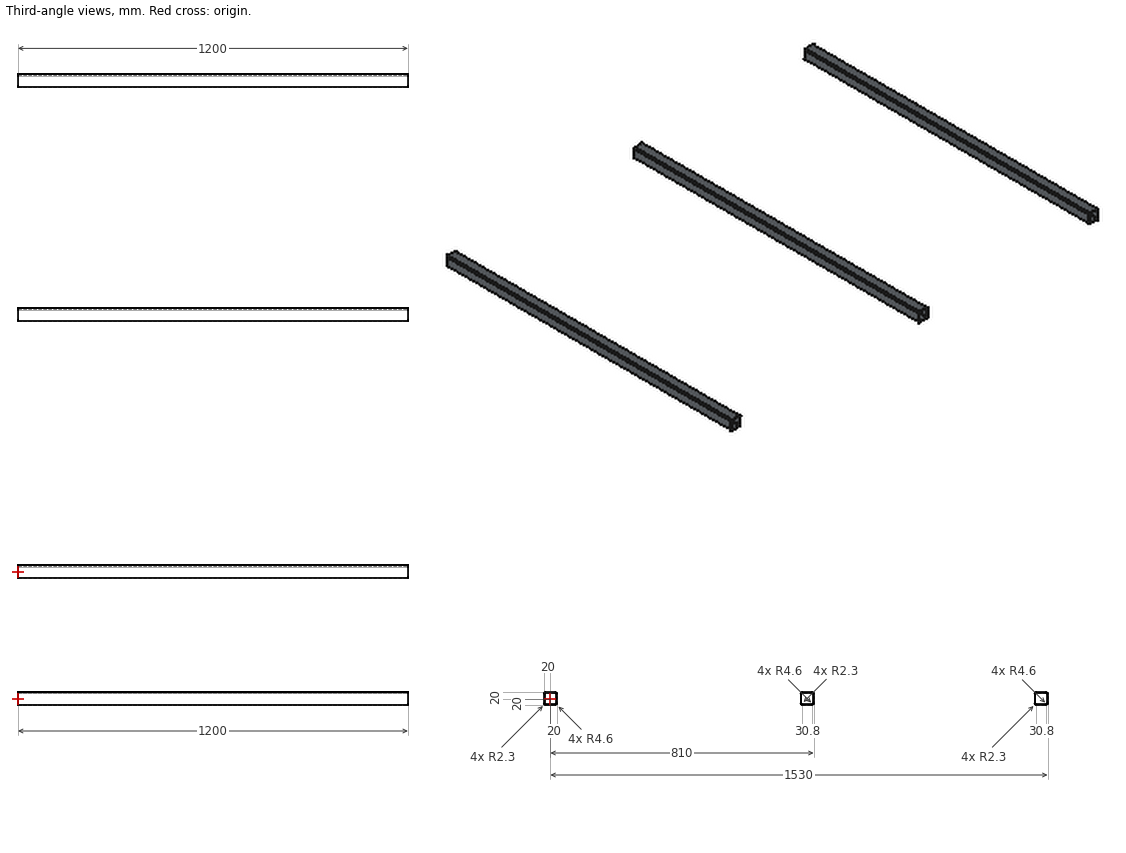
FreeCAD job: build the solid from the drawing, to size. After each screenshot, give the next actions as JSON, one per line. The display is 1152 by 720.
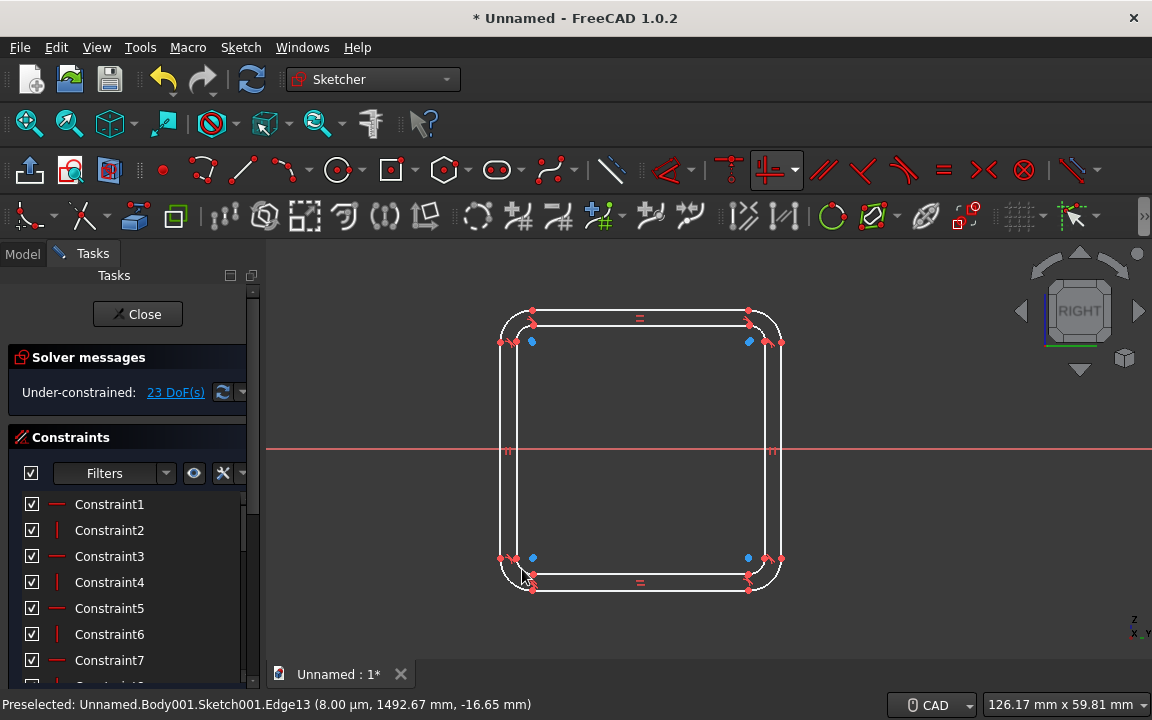
{"action": "left_click", "coordinate": [684, 574]}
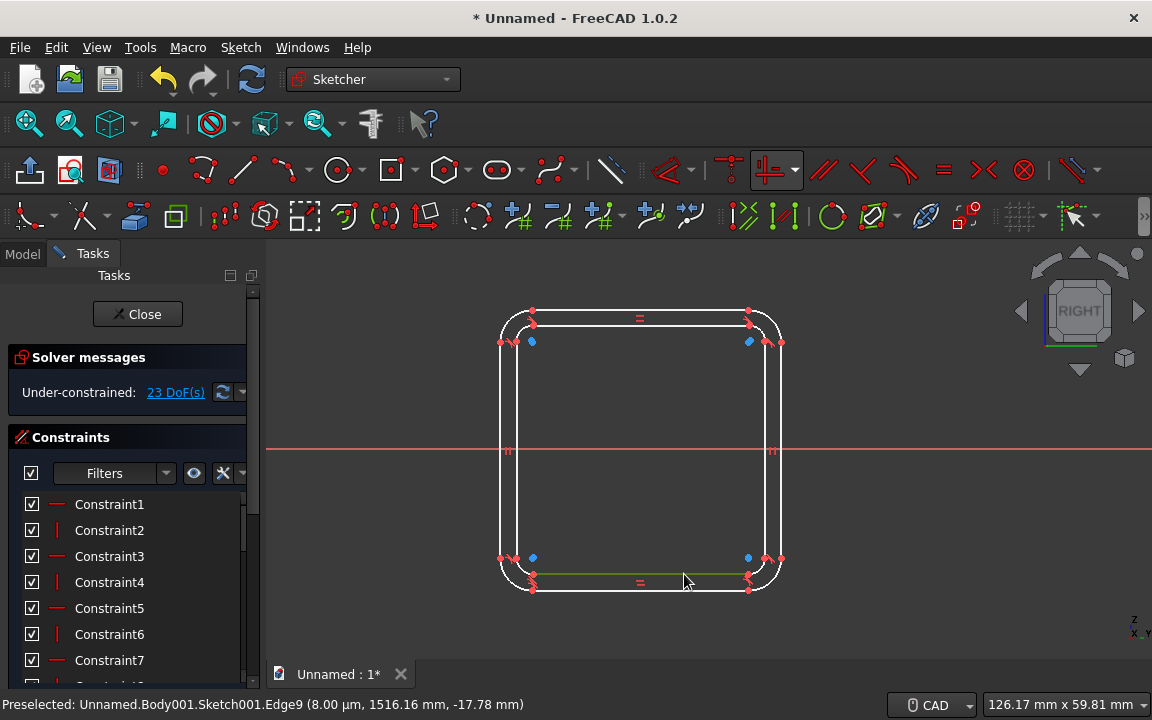
{"action": "left_click", "coordinate": [760, 570]}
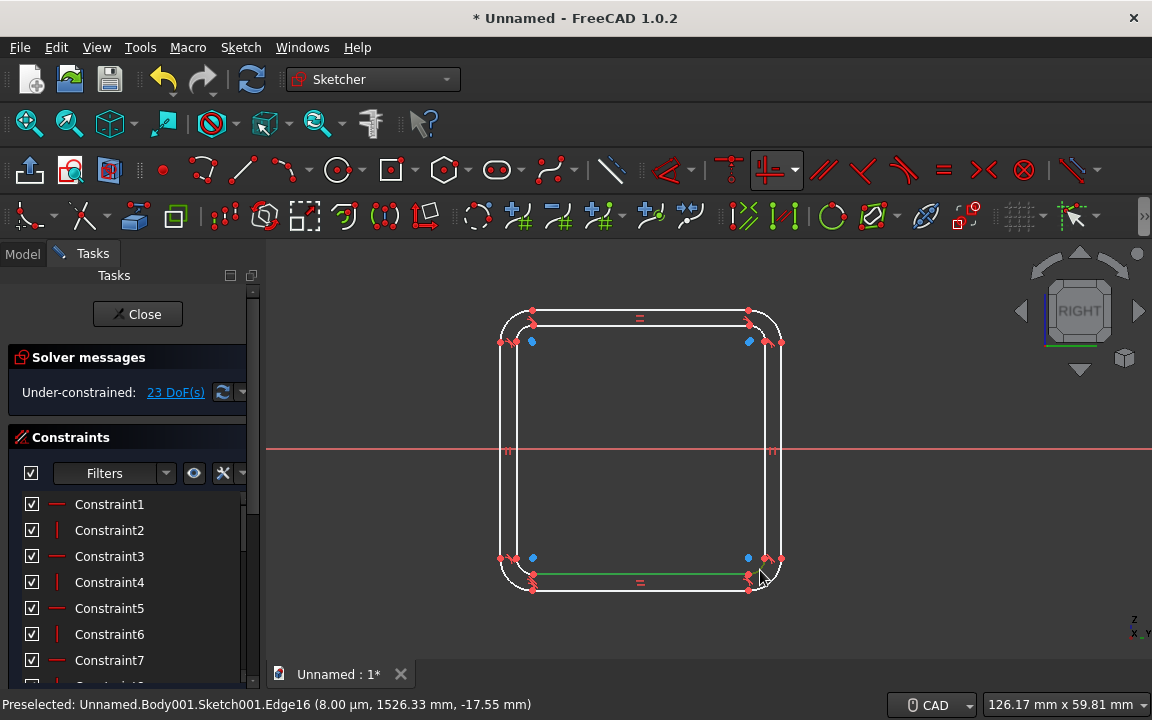
{"action": "key", "text": "t"}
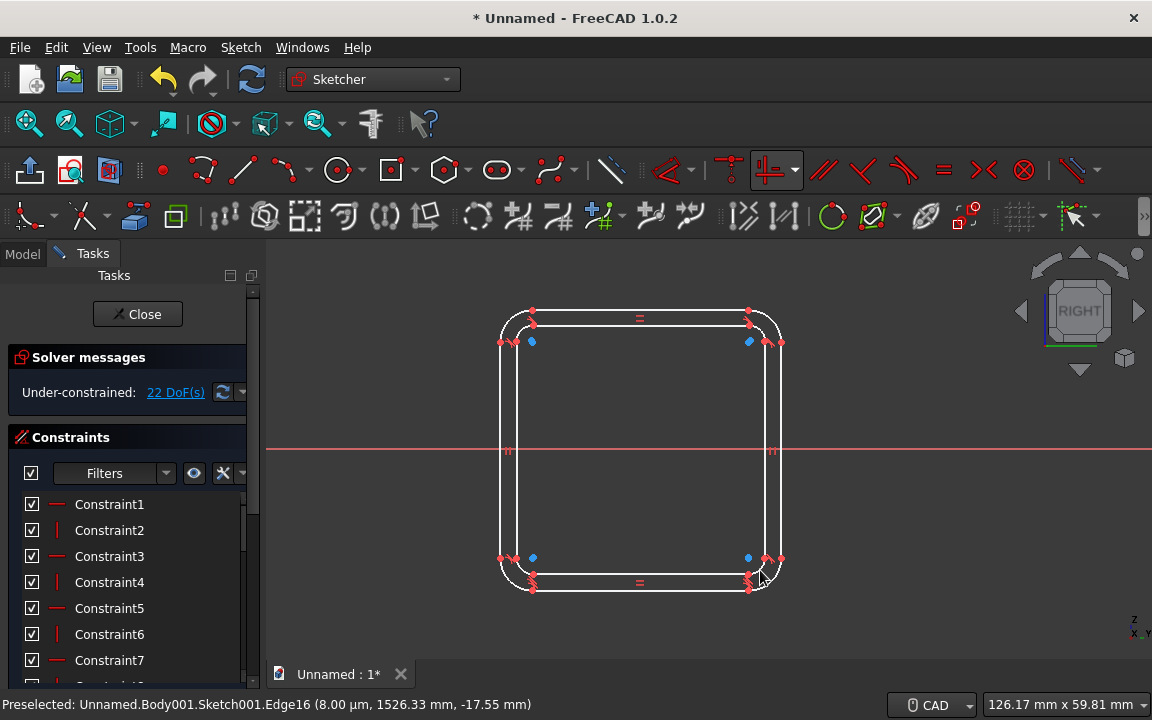
{"action": "left_click", "coordinate": [517, 493]}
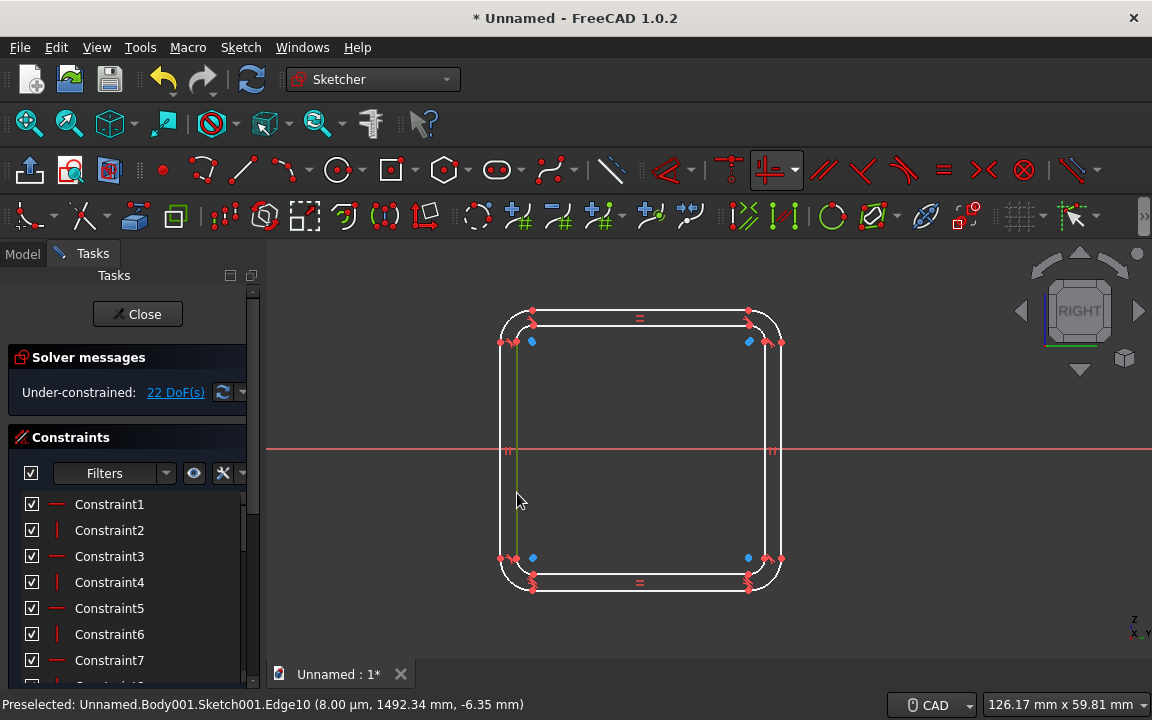
{"action": "left_click", "coordinate": [522, 570]}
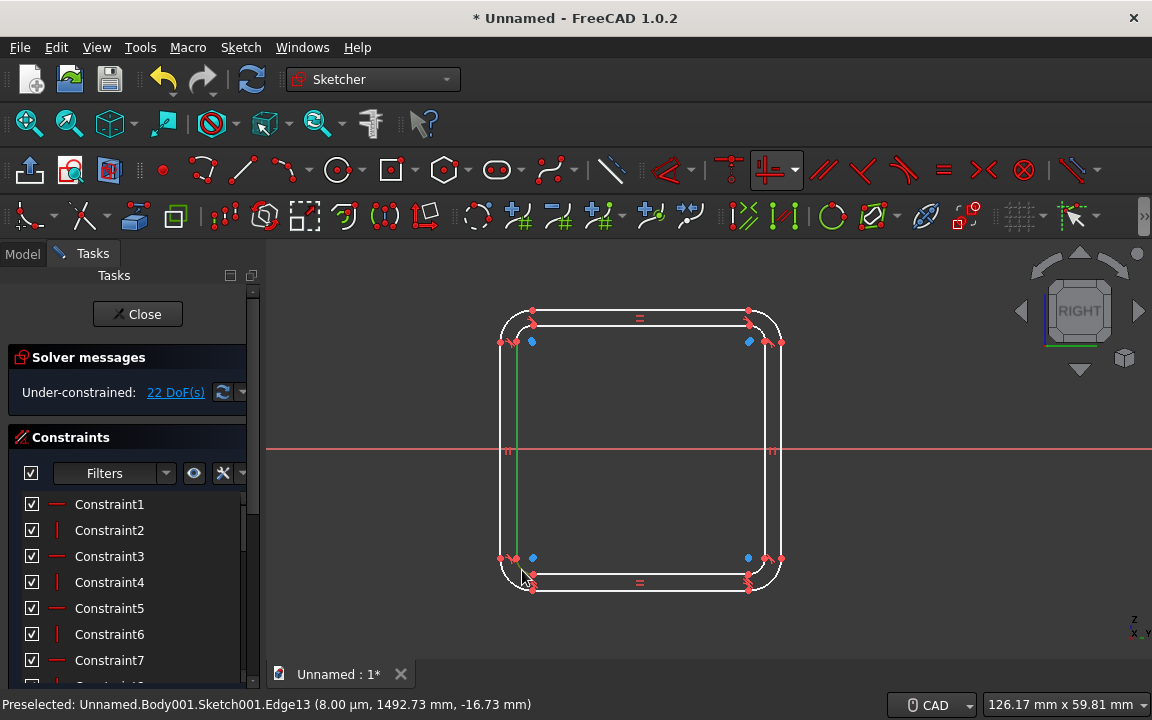
{"action": "key", "text": "t"}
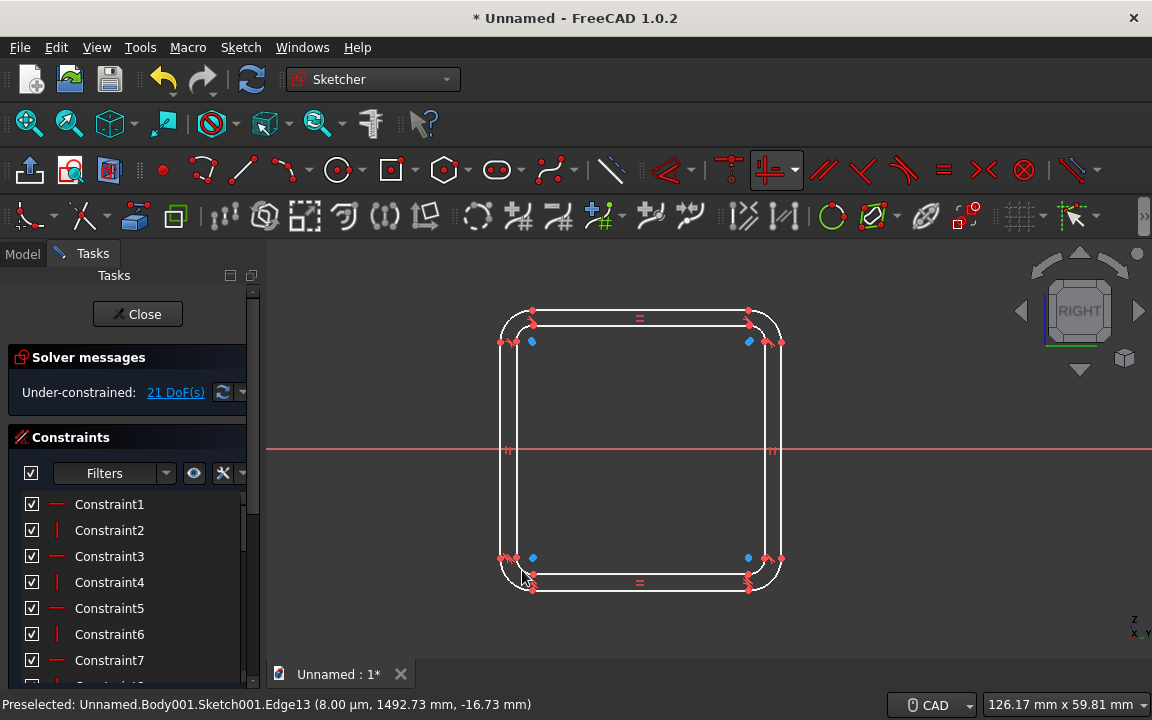
{"action": "left_click", "coordinate": [517, 493]}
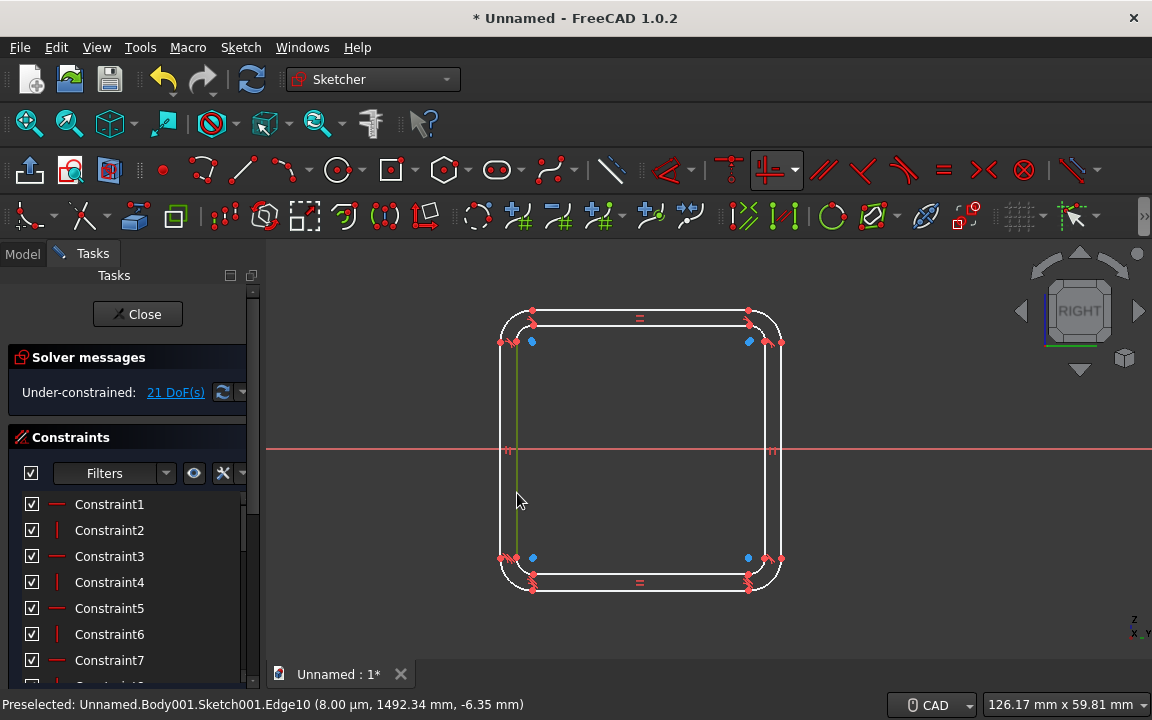
{"action": "left_click", "coordinate": [521, 330]}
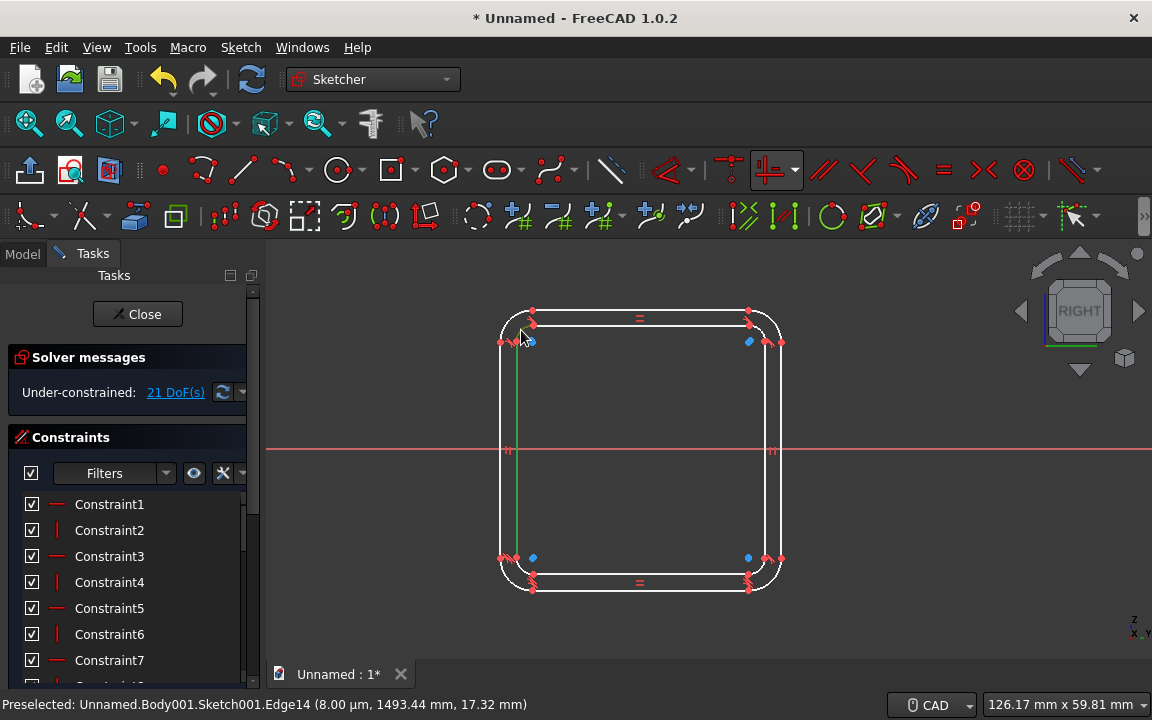
{"action": "key", "text": "t"}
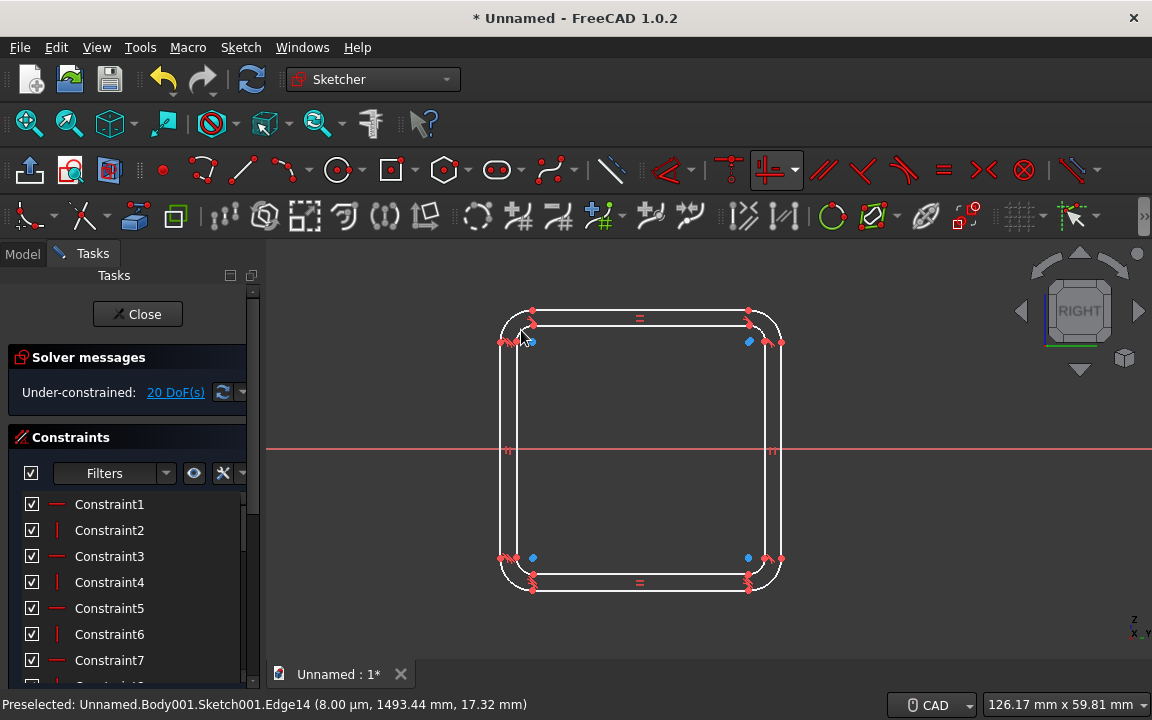
{"action": "left_click", "coordinate": [598, 326]}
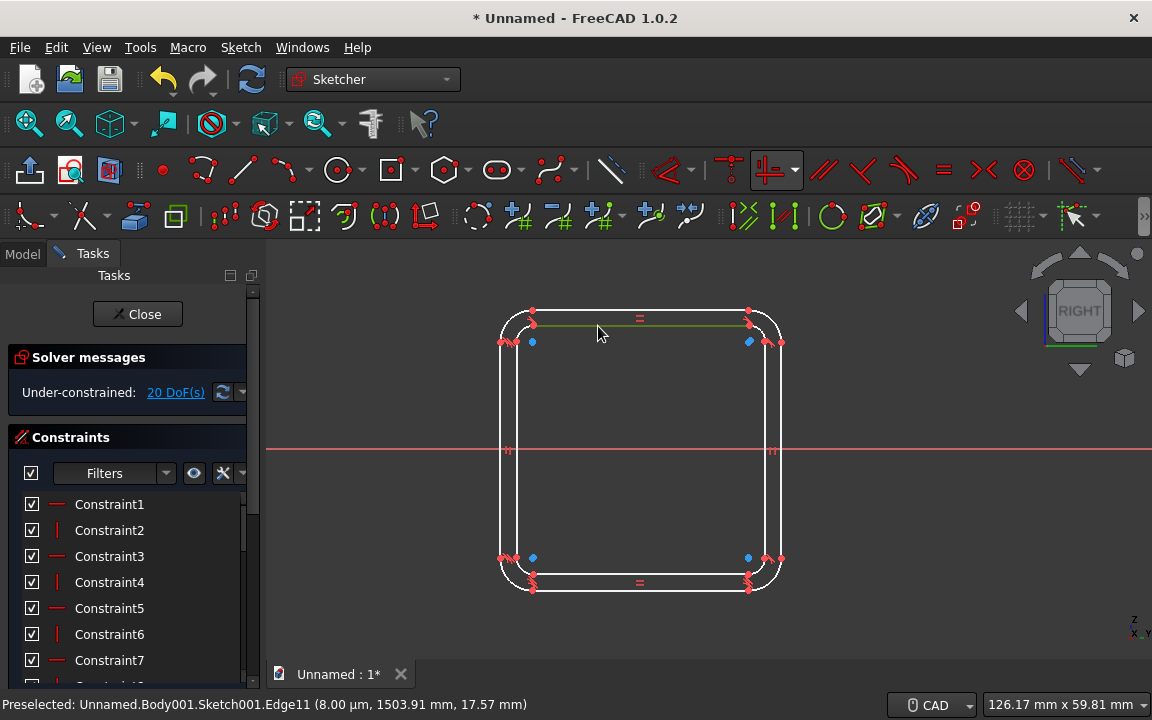
{"action": "left_click", "coordinate": [522, 331]}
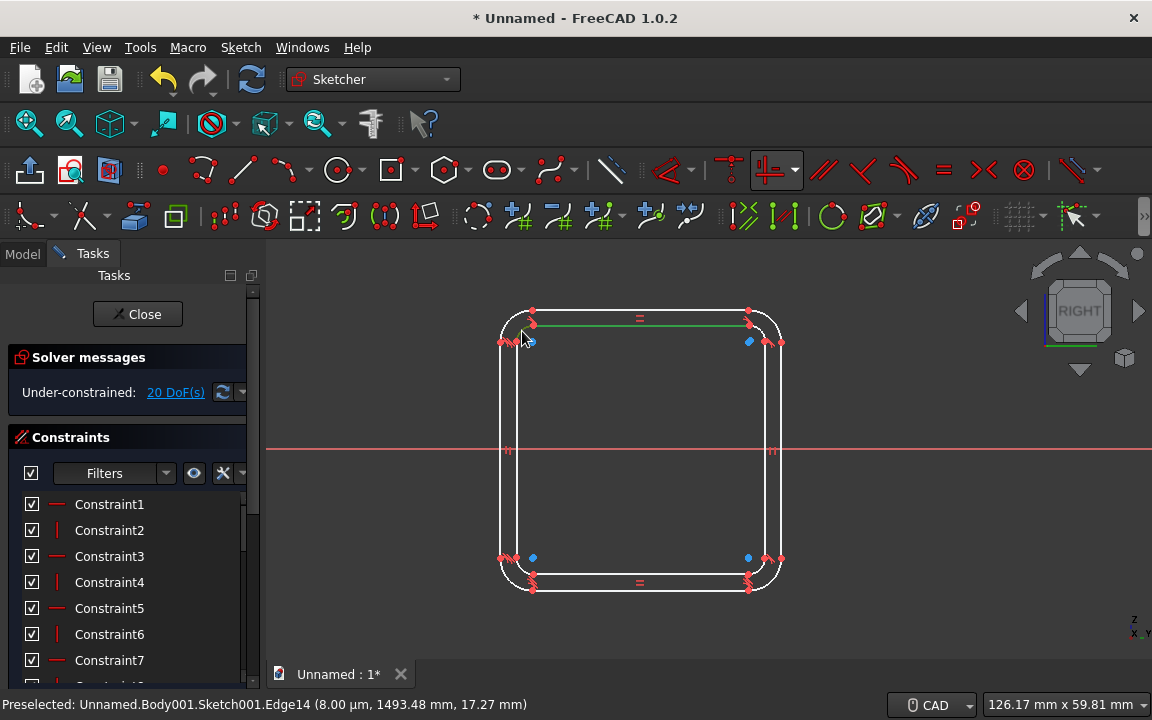
{"action": "key", "text": "t"}